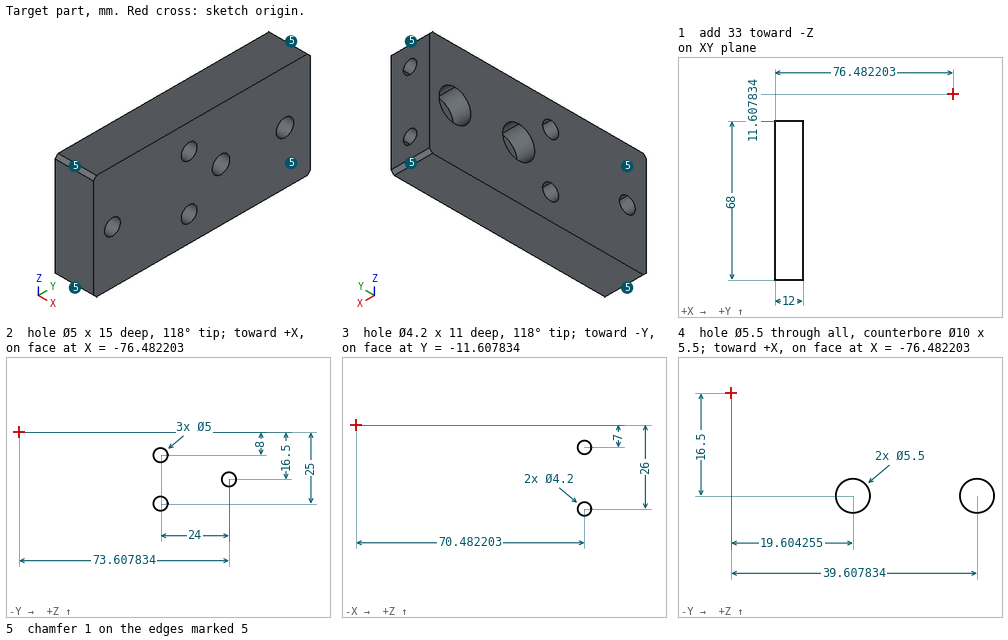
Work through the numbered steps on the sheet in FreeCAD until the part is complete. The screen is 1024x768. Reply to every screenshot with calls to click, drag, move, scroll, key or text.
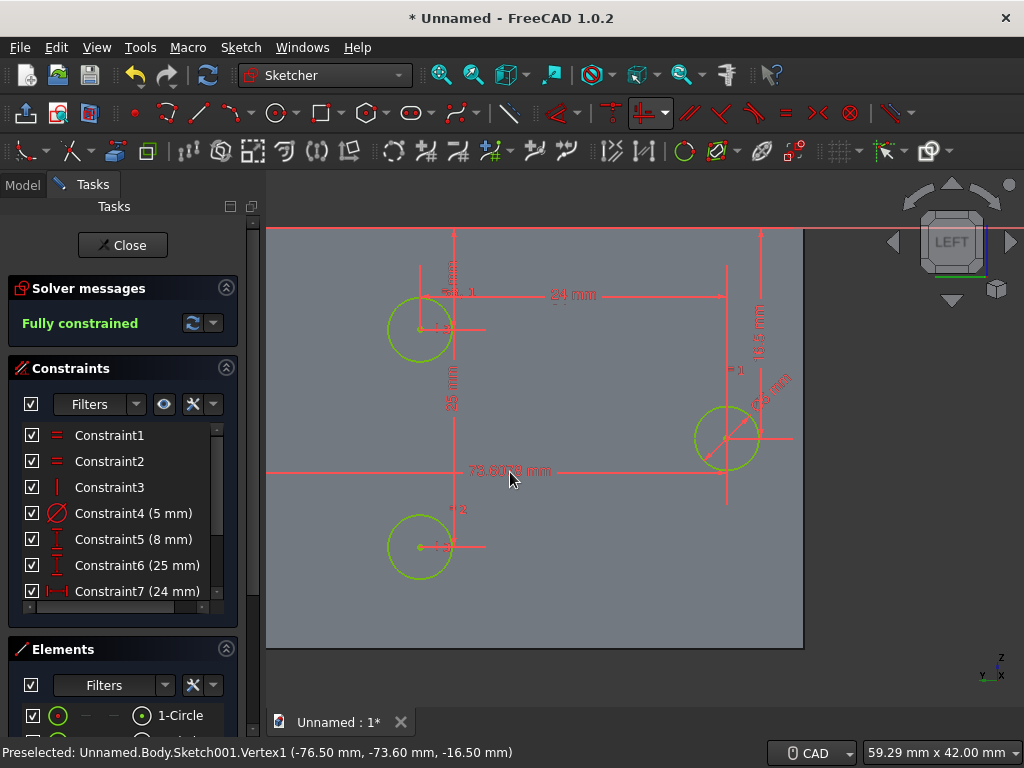
click(123, 245)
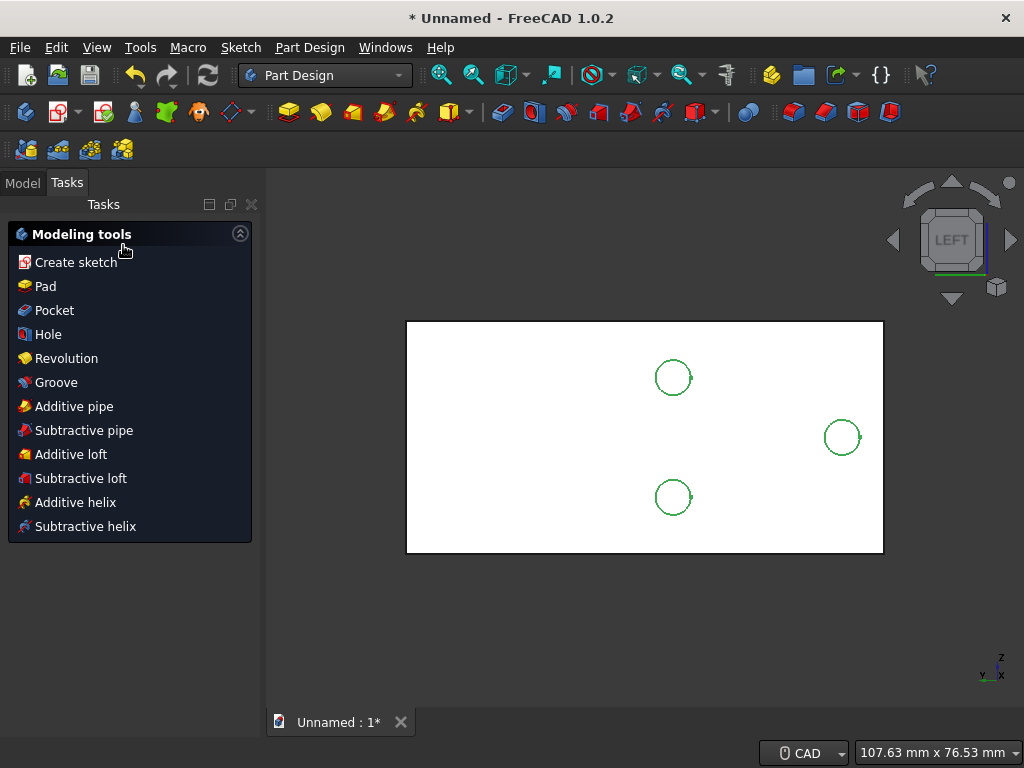
click(536, 112)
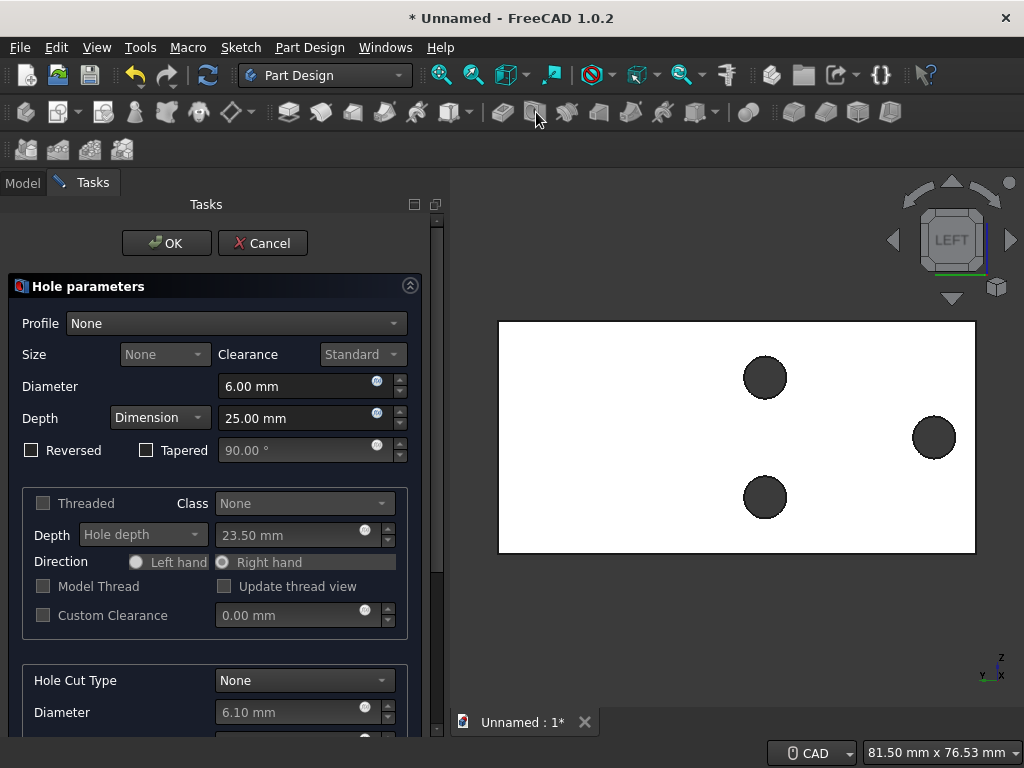
triple_click(305, 386)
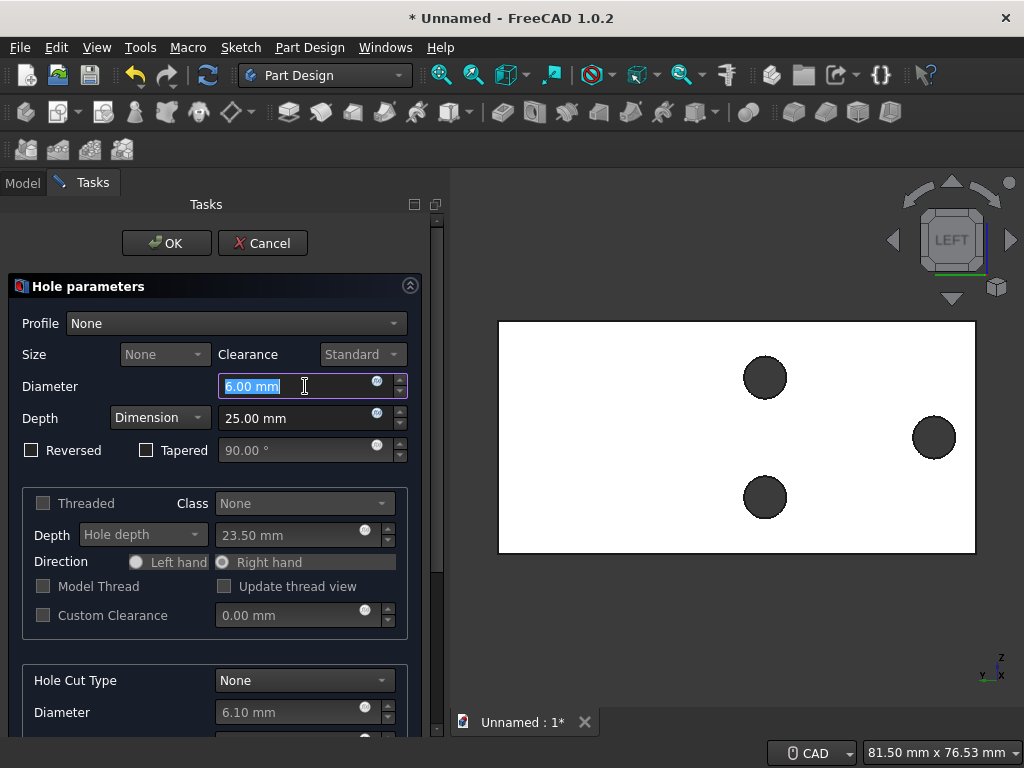
text(5)
key(Tab)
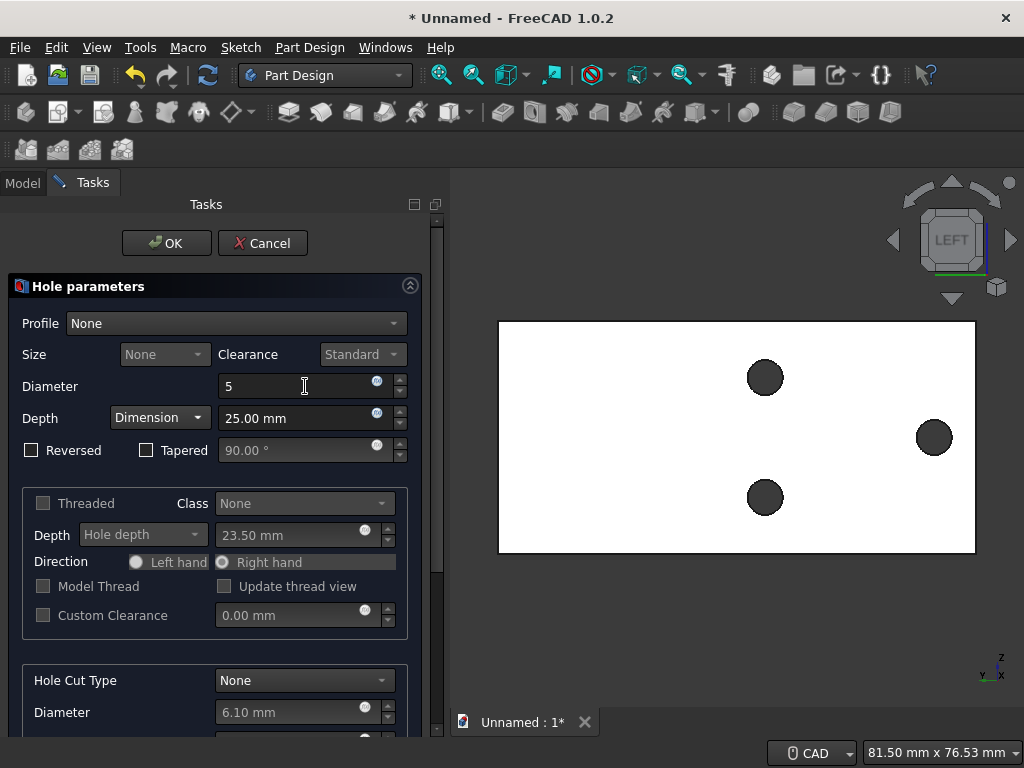
triple_click(305, 418)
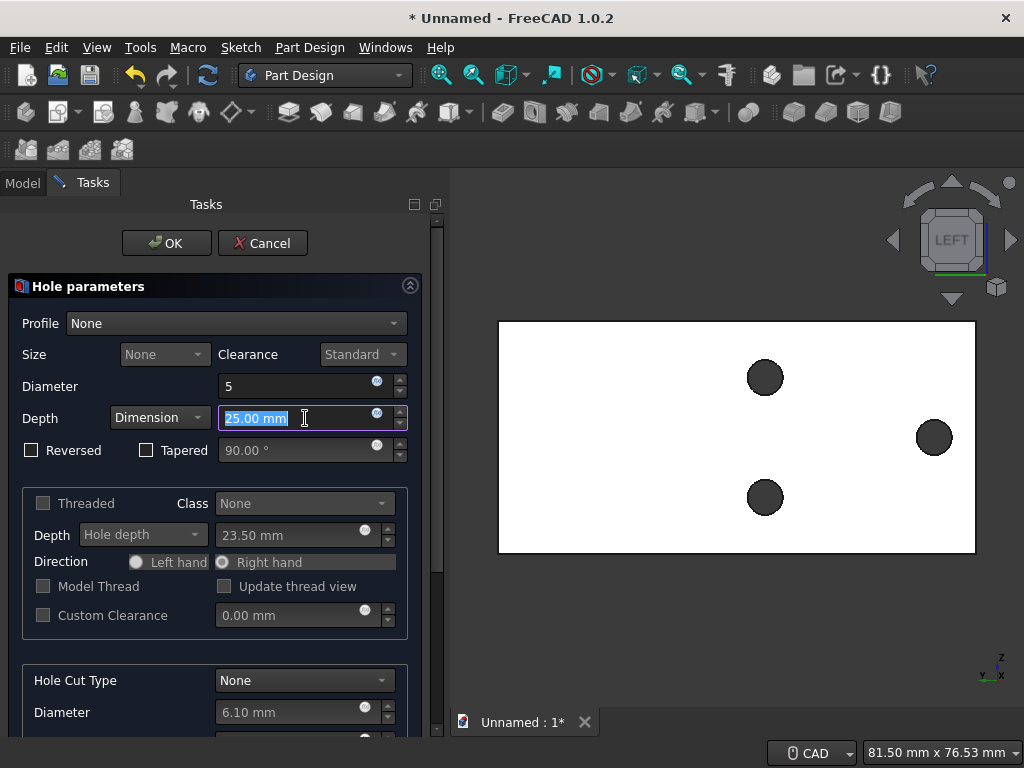
text(15)
key(Tab)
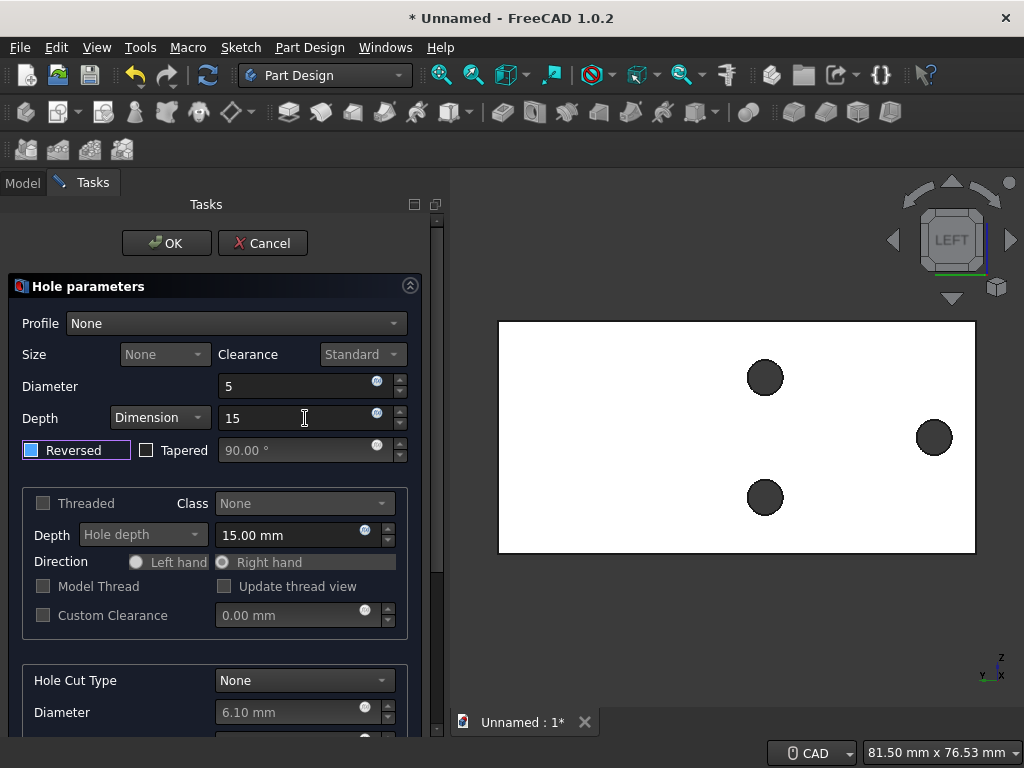
click(167, 243)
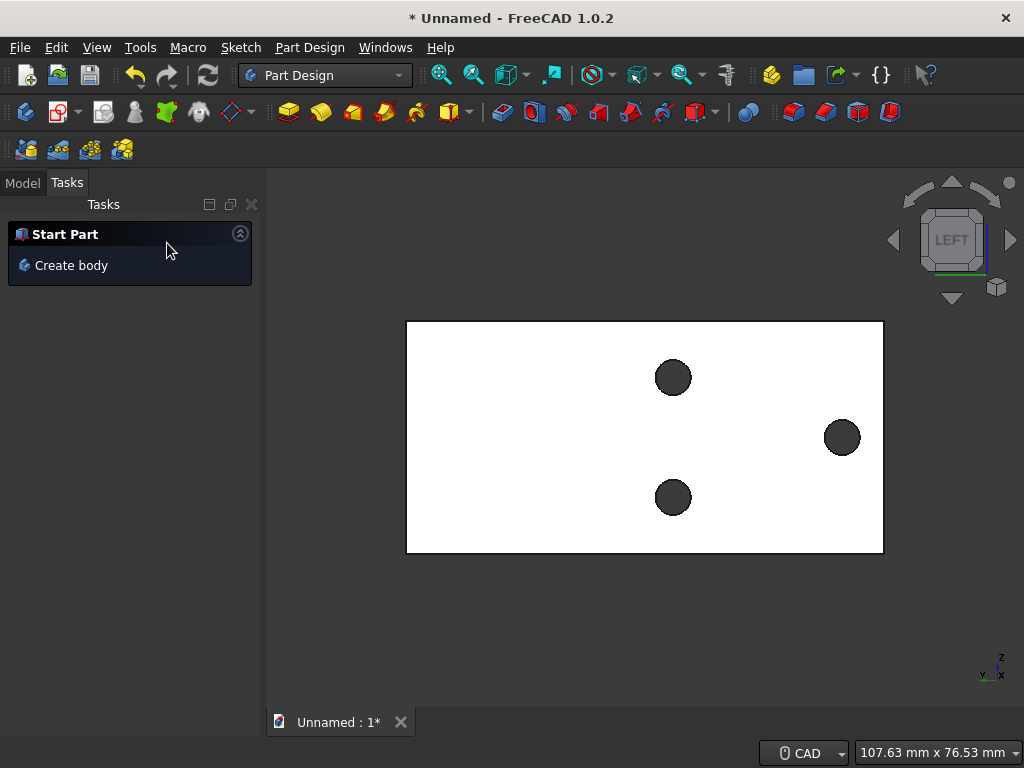
key(4)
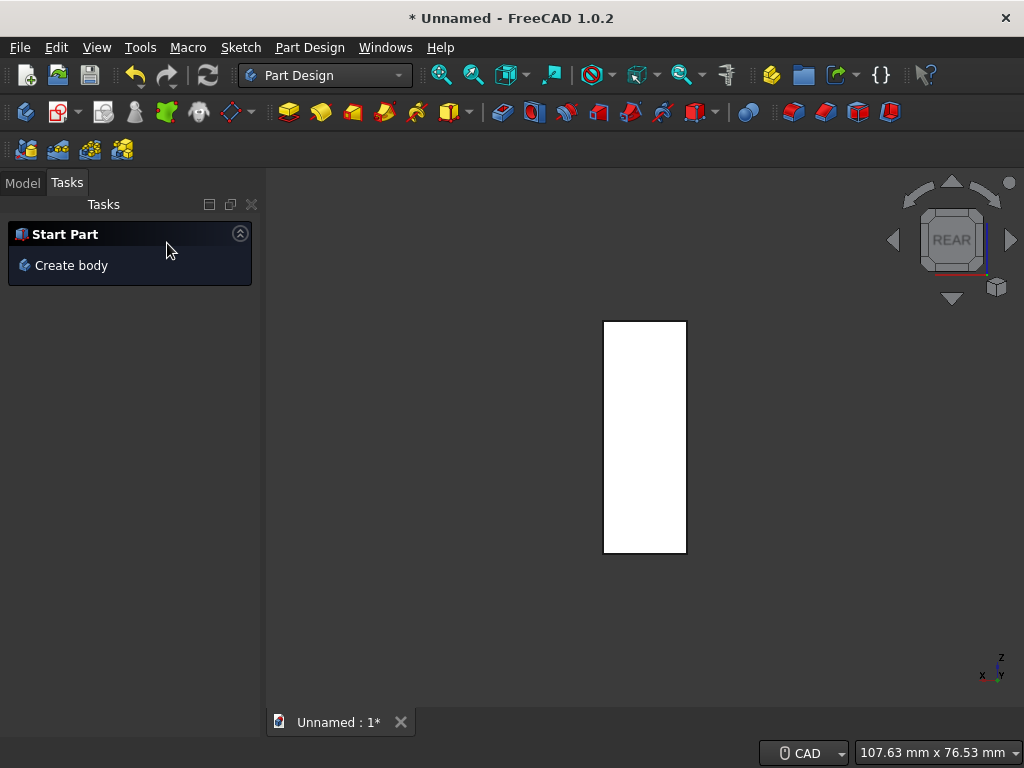
click(442, 76)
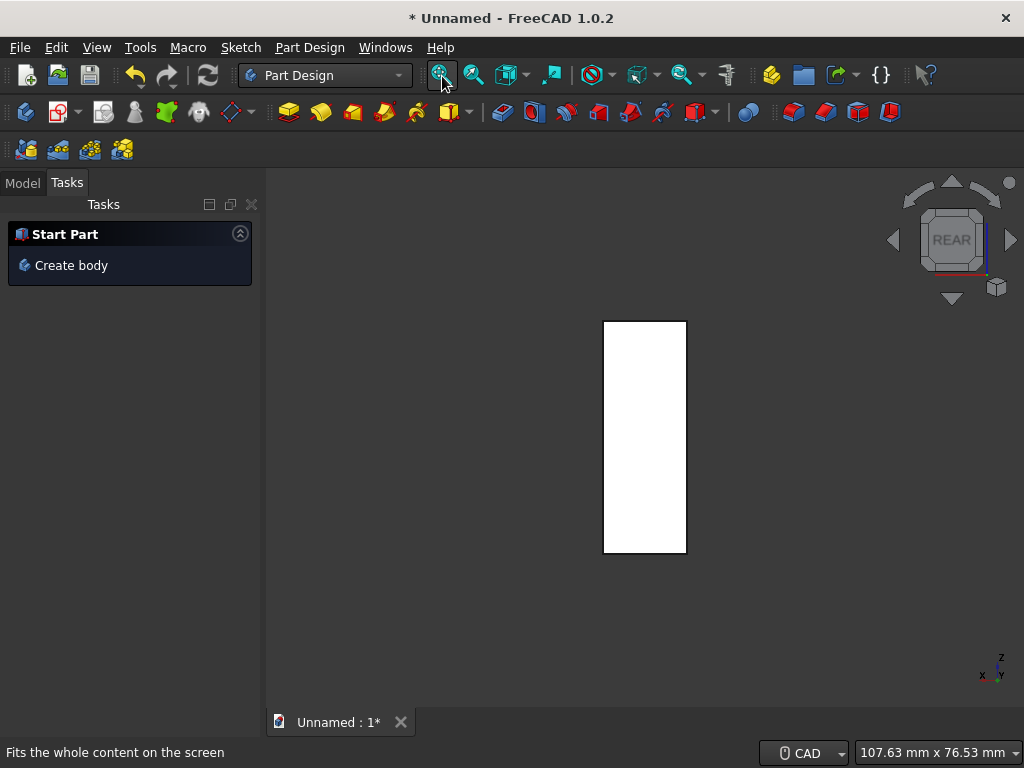
click(645, 370)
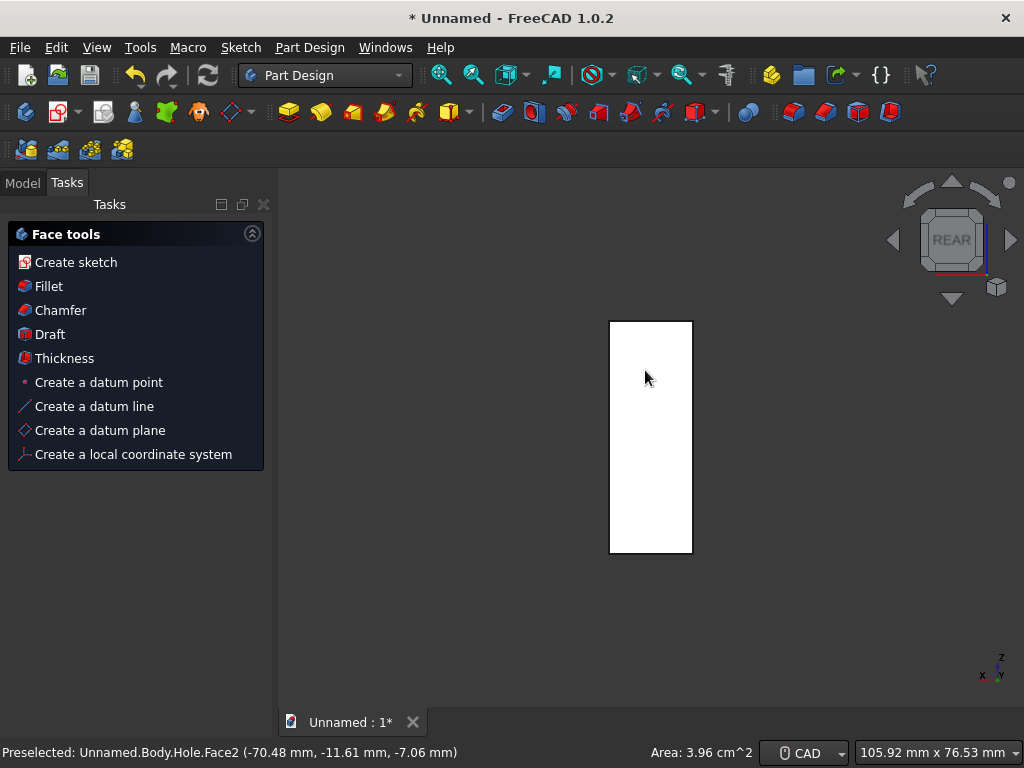
click(58, 112)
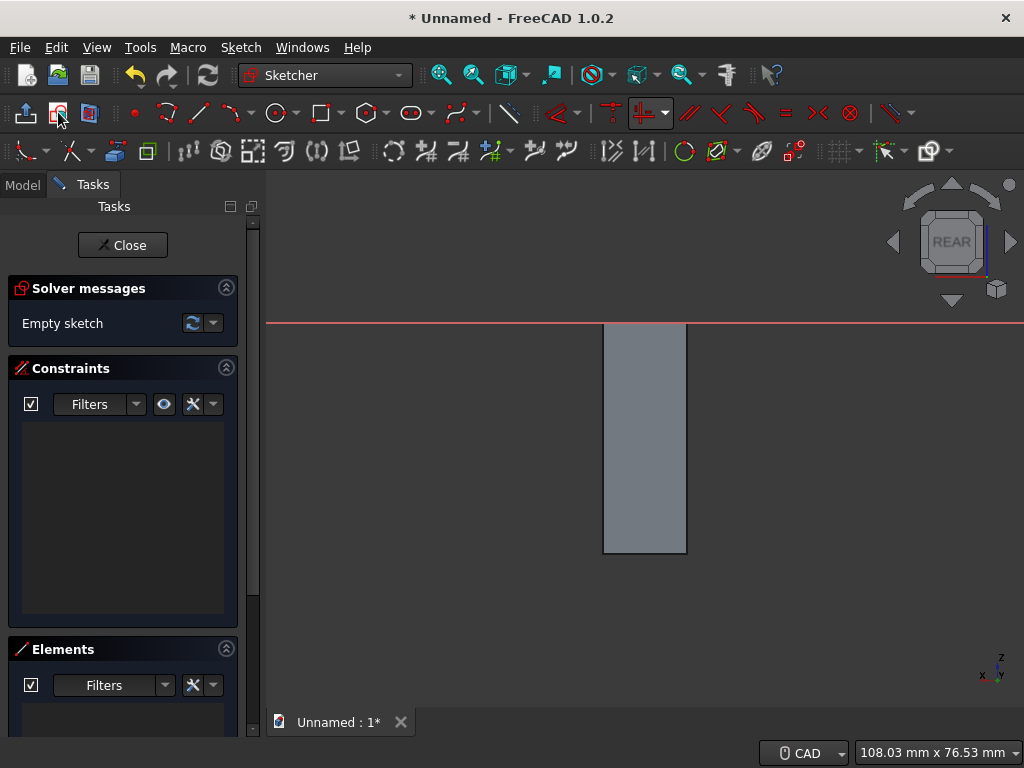
scroll(701, 439, up, 4)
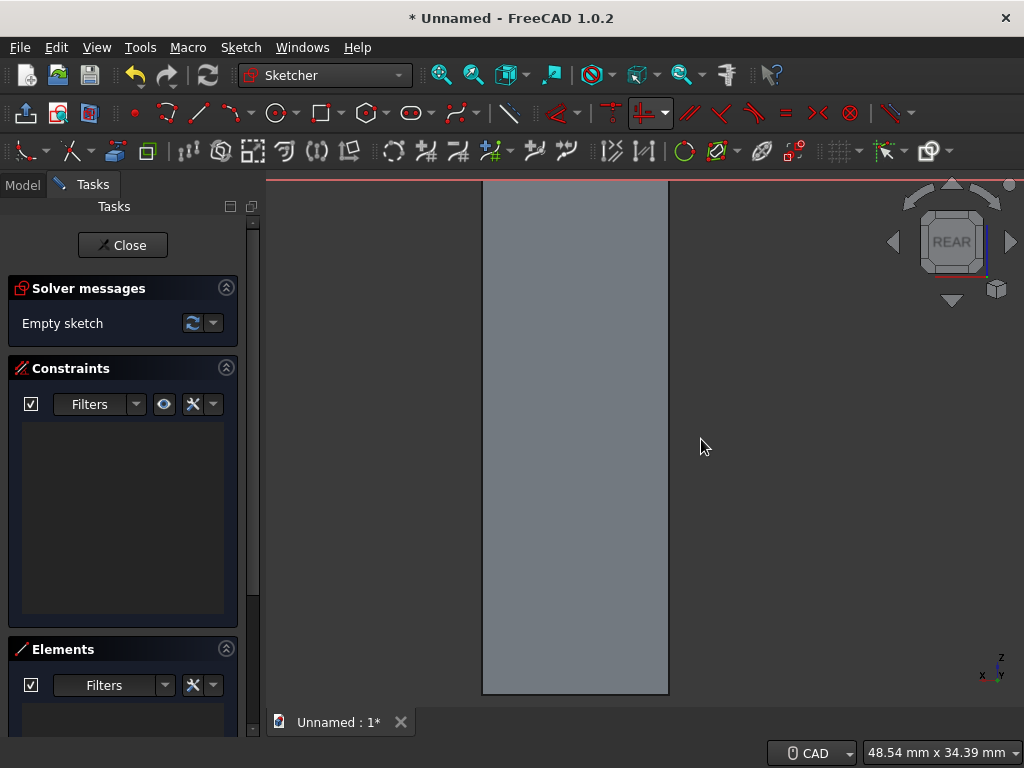
click(276, 114)